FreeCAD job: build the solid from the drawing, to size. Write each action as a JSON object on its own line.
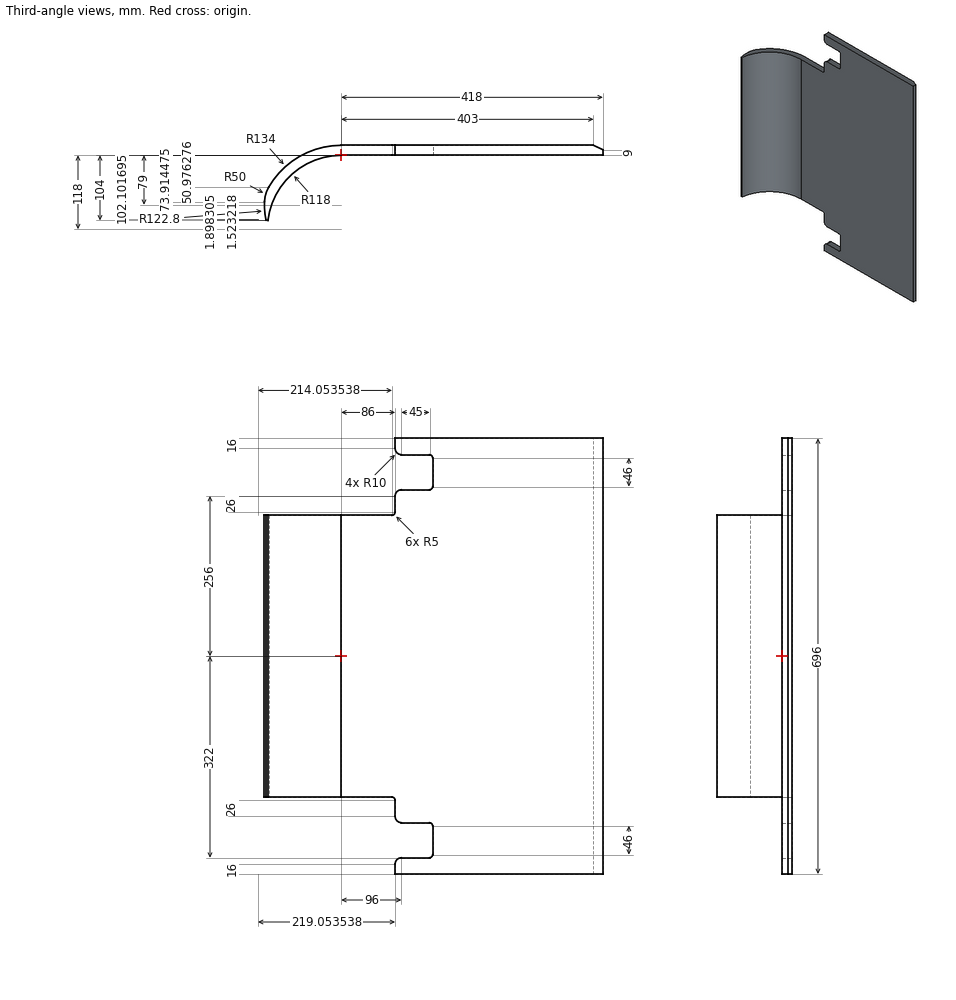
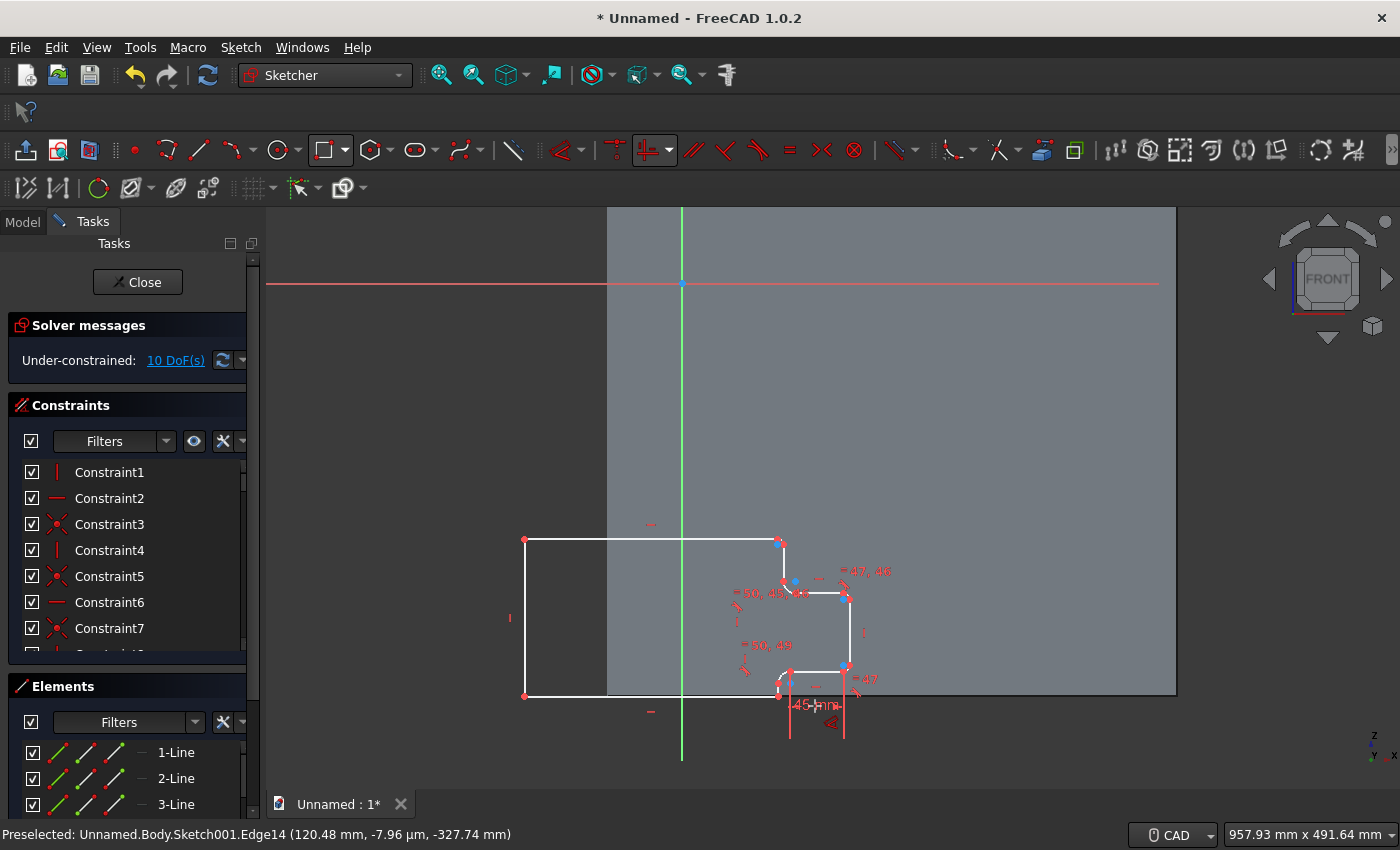
{"action": "scroll", "coordinate": [778, 690], "scroll_direction": "up", "scroll_amount": 4}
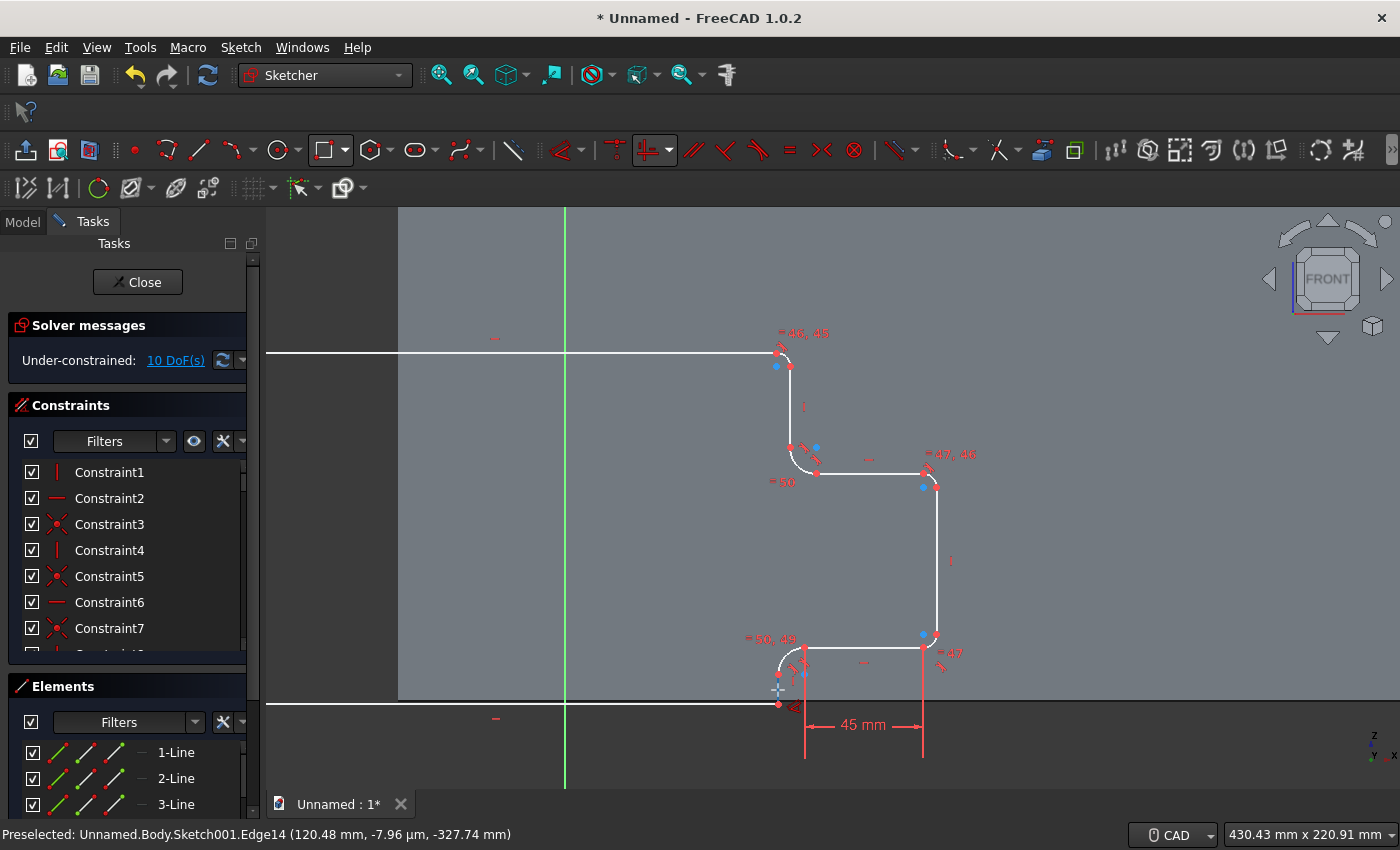
{"action": "left_click", "coordinate": [779, 689]}
{"action": "left_click", "coordinate": [813, 689]}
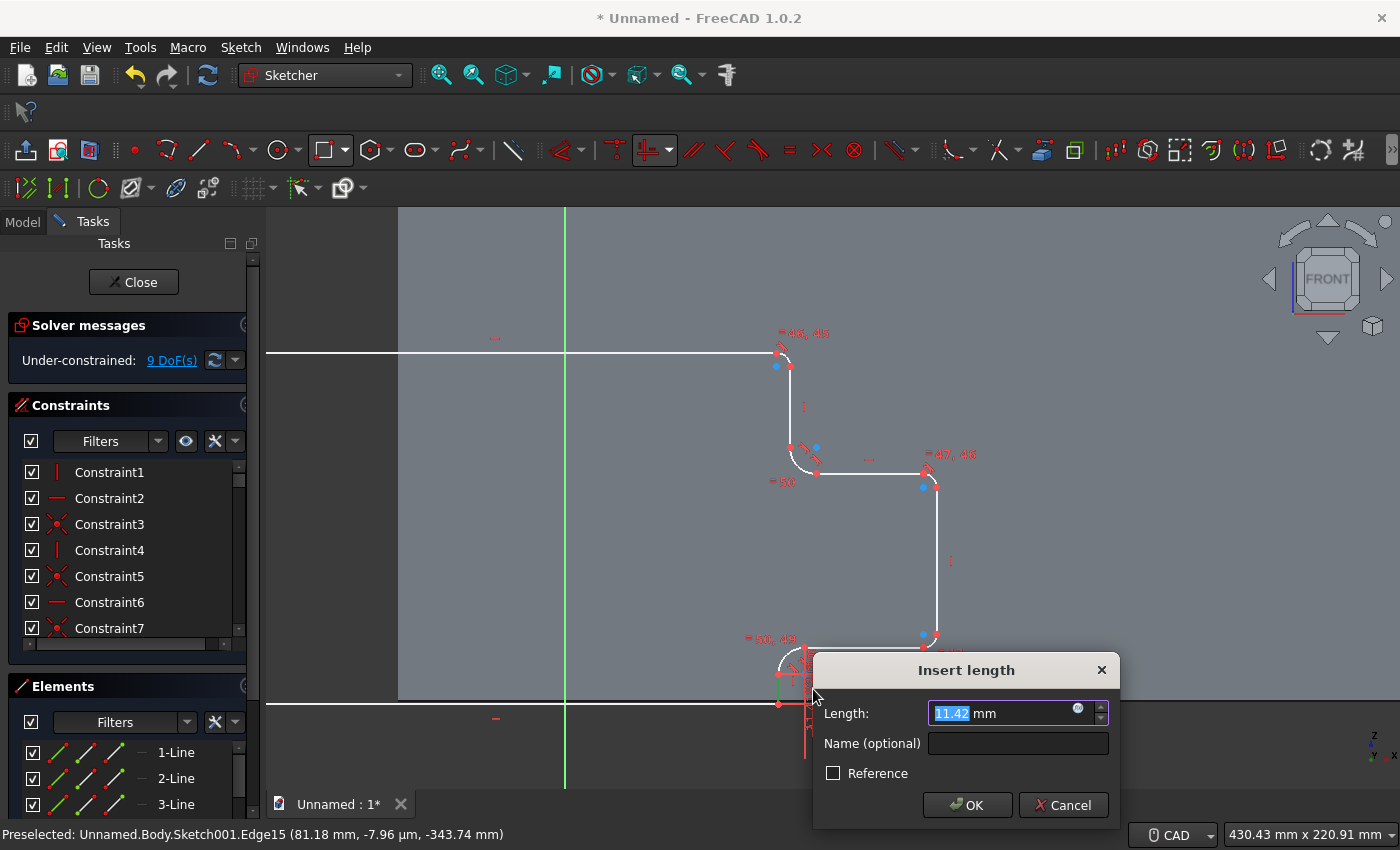
{"action": "type", "text": "16"}
{"action": "key", "text": "Return"}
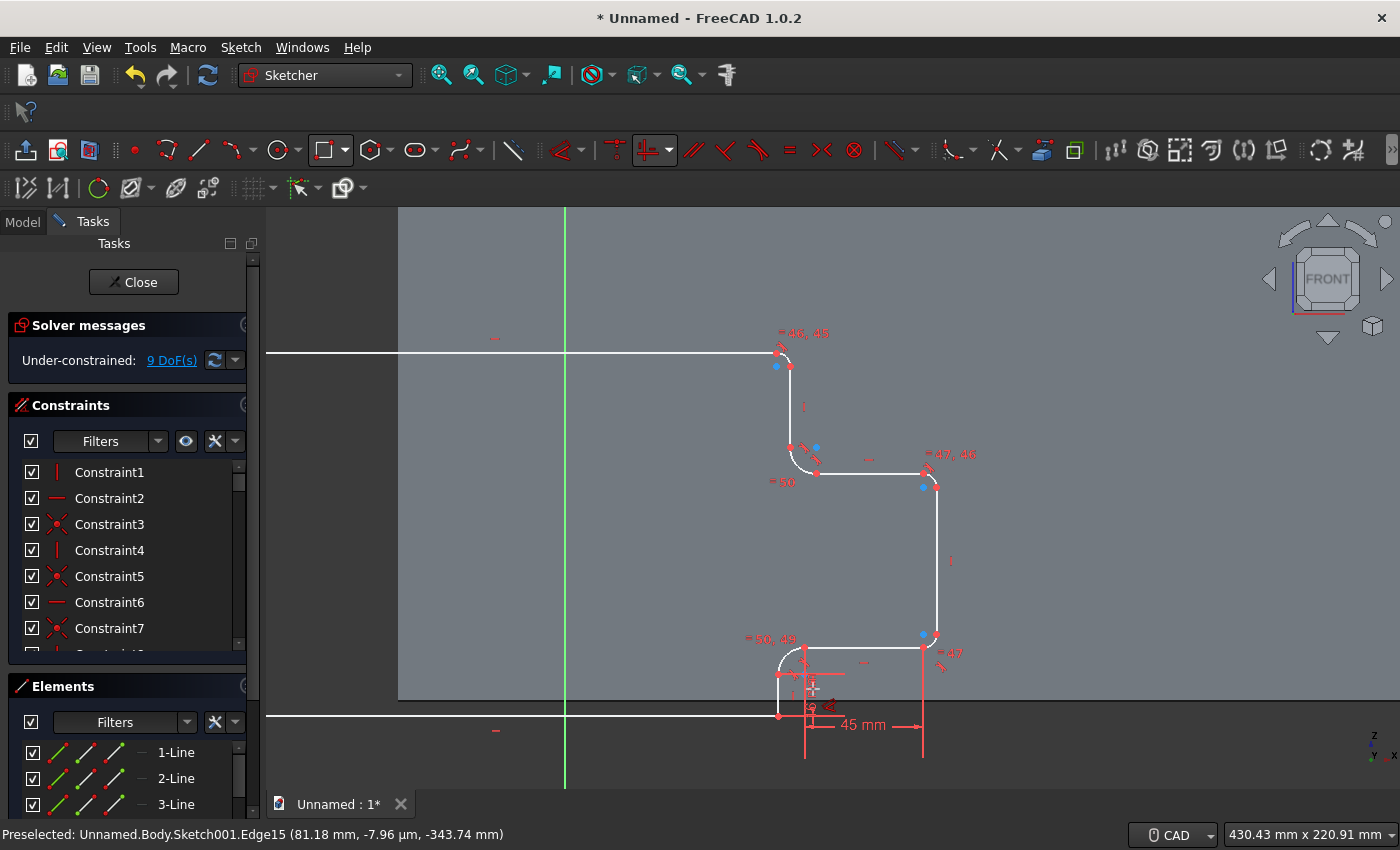
{"action": "left_click", "coordinate": [790, 391]}
{"action": "left_click", "coordinate": [824, 407]}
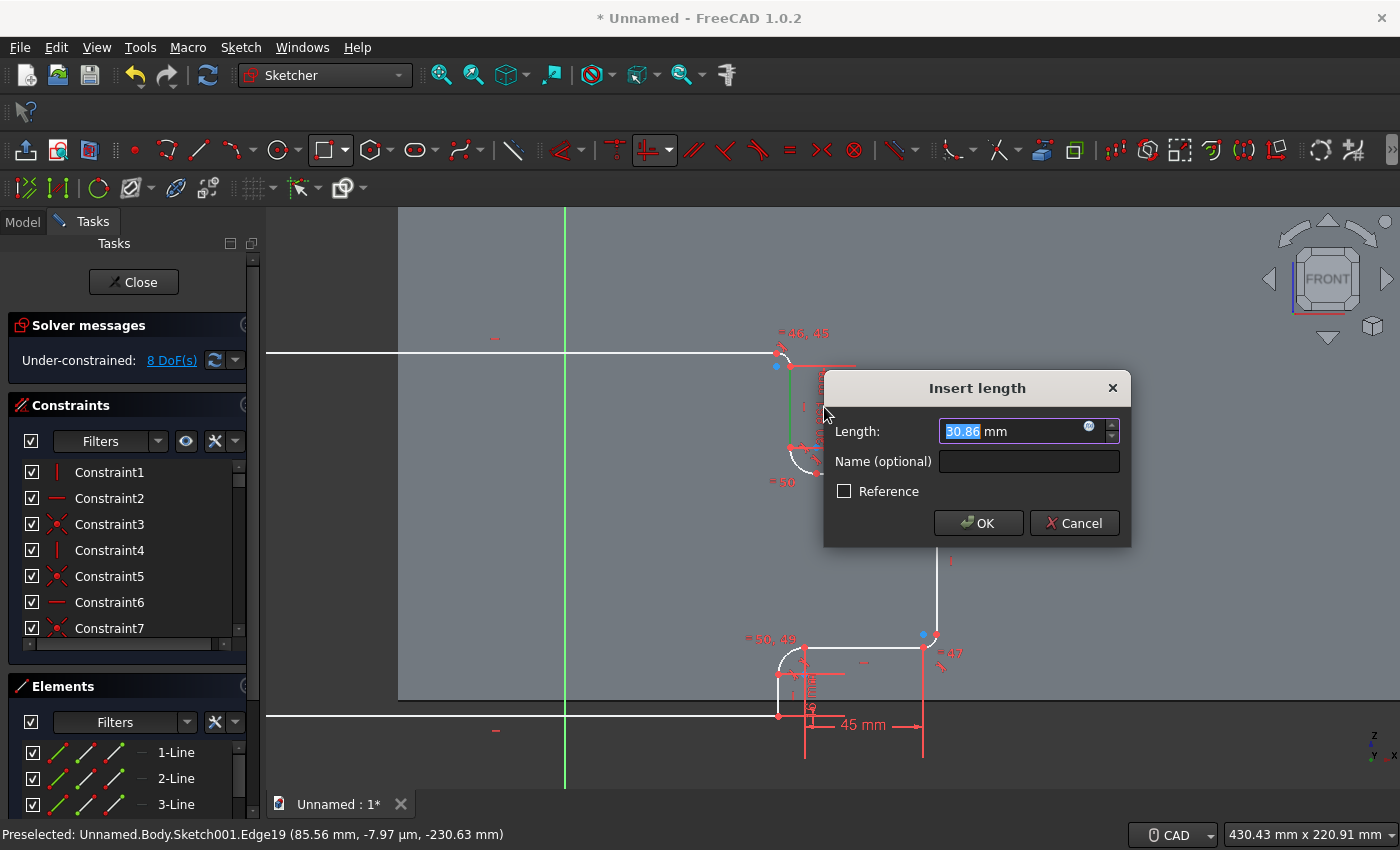
{"action": "type", "text": "26"}
{"action": "key", "text": "Return"}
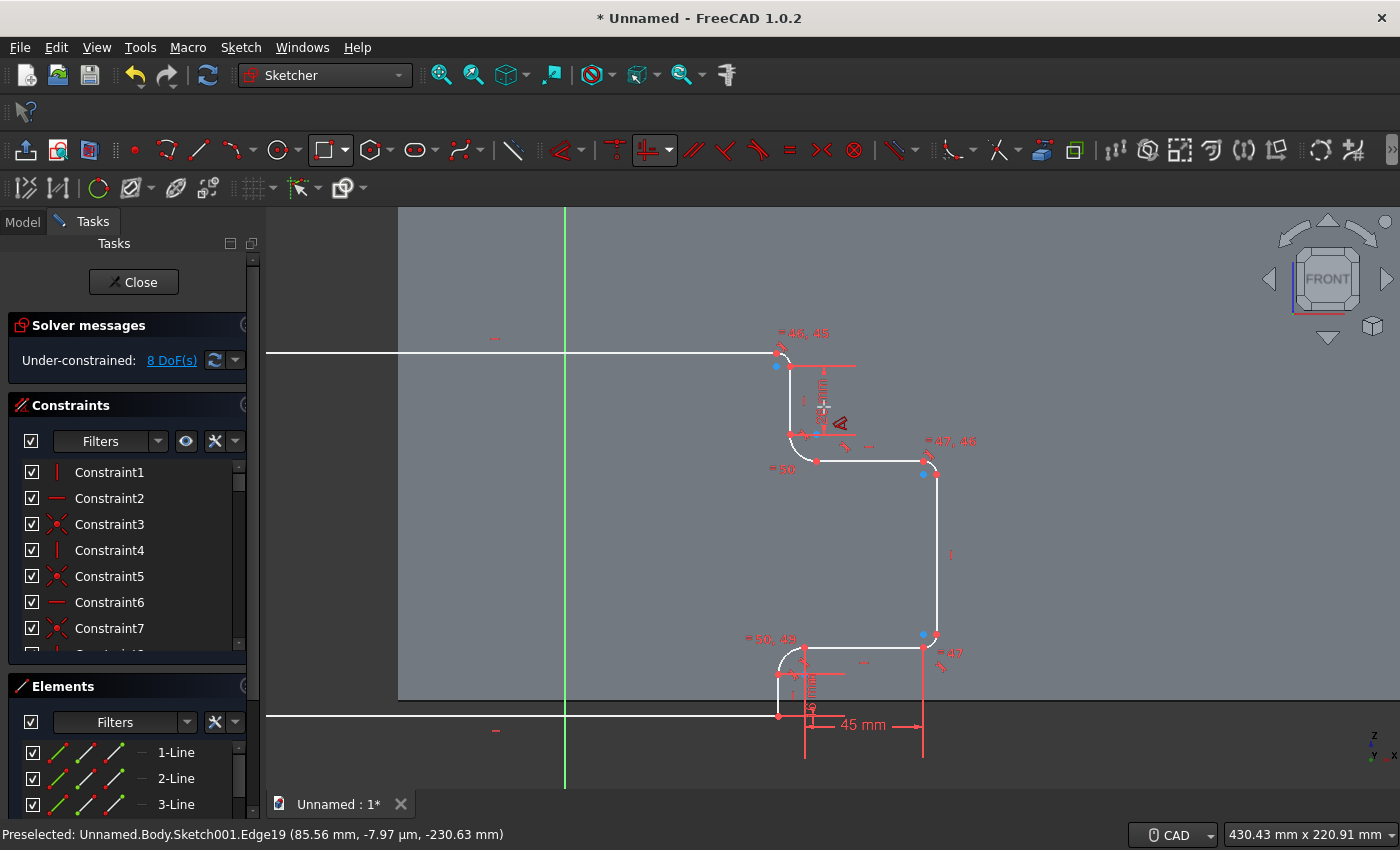
{"action": "left_click", "coordinate": [848, 461]}
{"action": "left_click", "coordinate": [870, 495]}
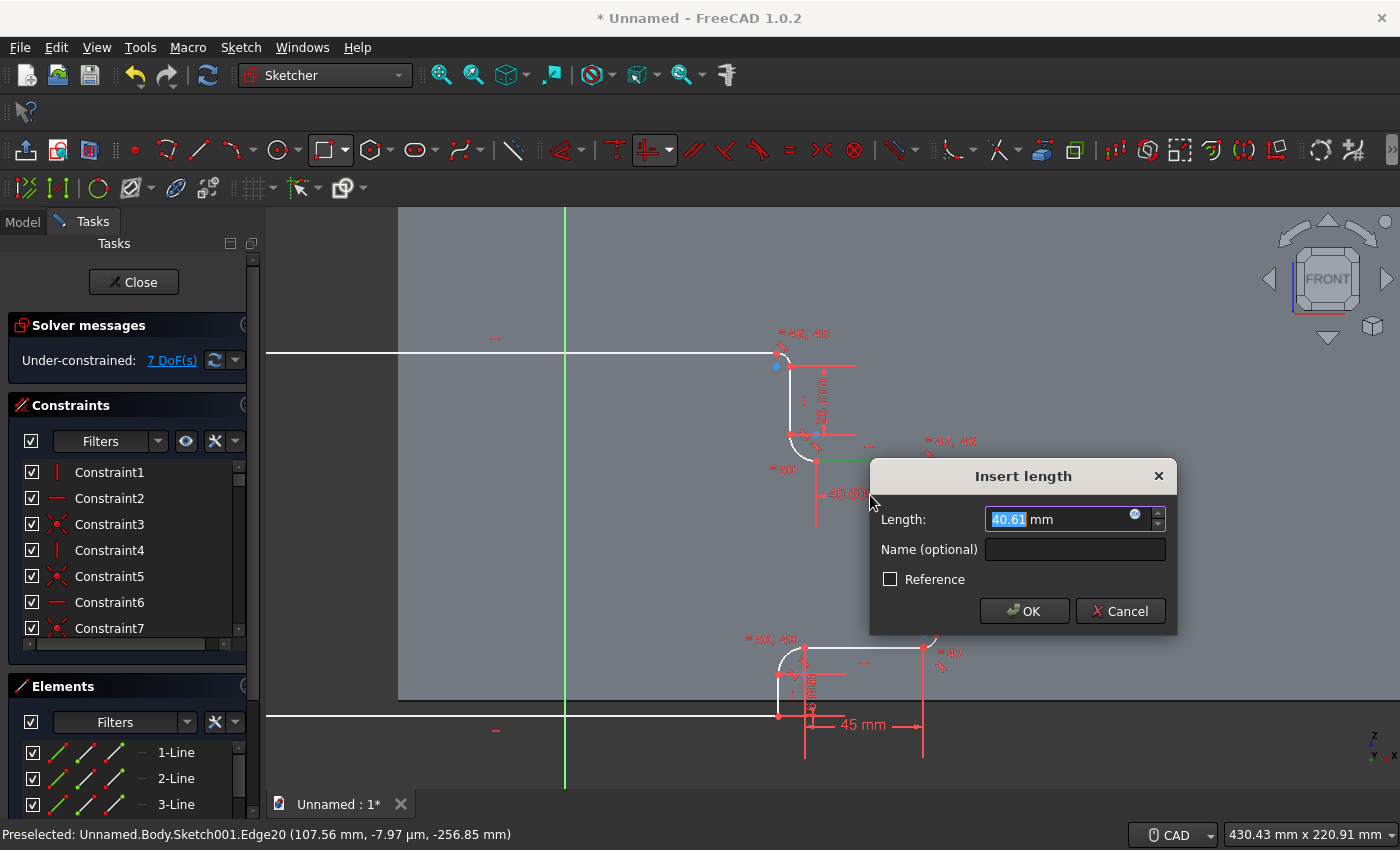
{"action": "type", "text": "45"}
{"action": "key", "text": "Return"}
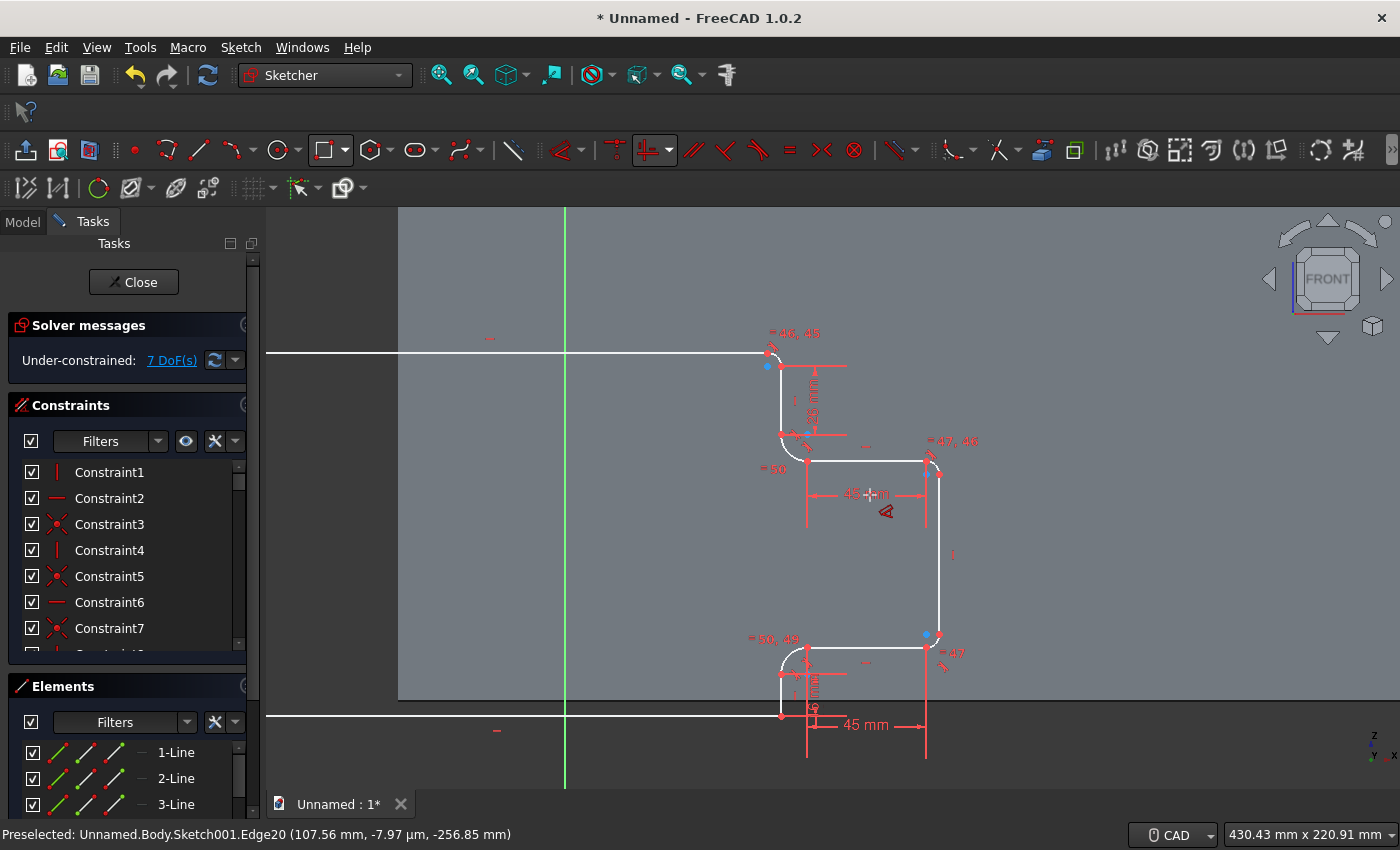
{"action": "scroll", "coordinate": [811, 679], "scroll_direction": "down", "scroll_amount": 8}